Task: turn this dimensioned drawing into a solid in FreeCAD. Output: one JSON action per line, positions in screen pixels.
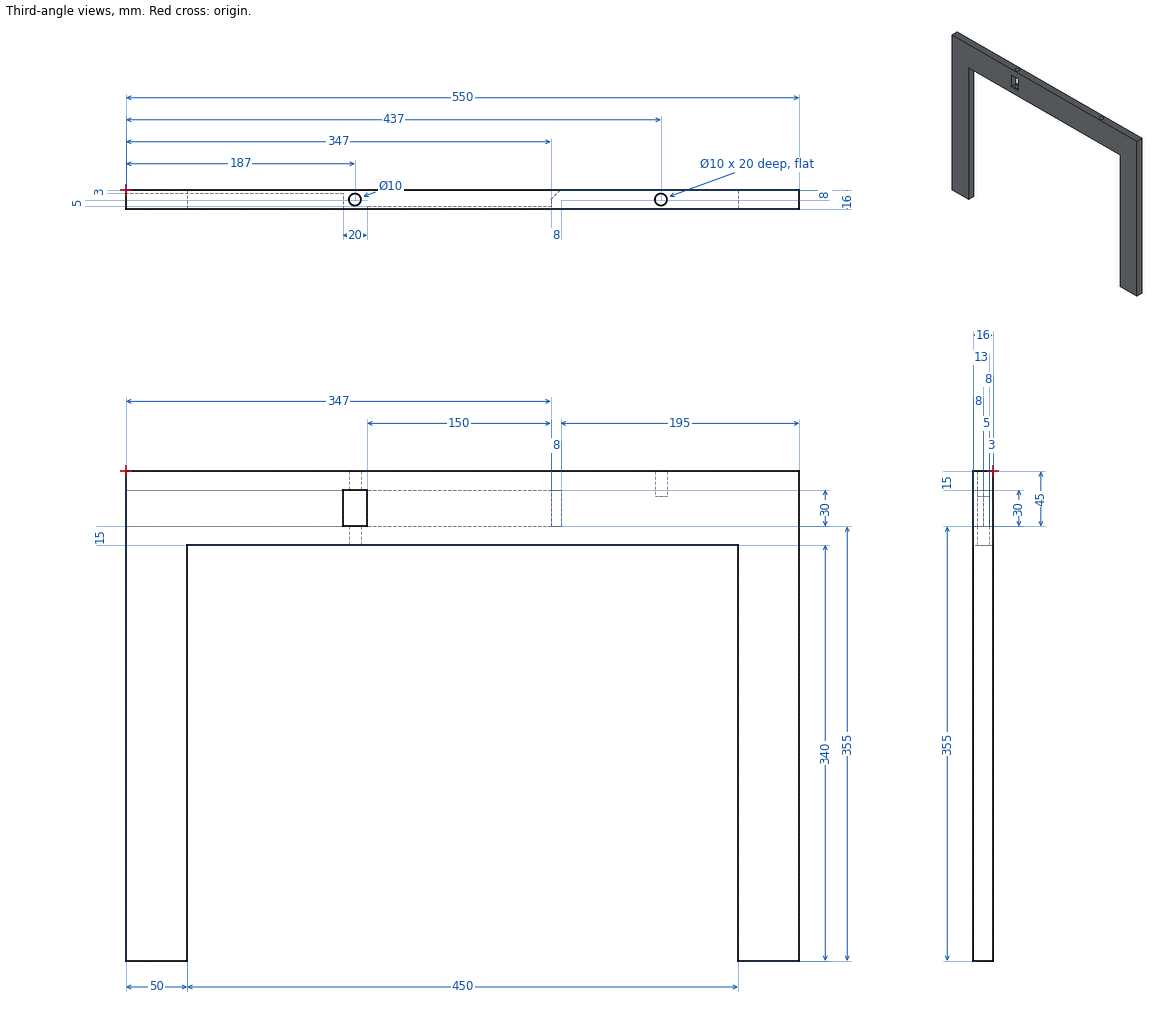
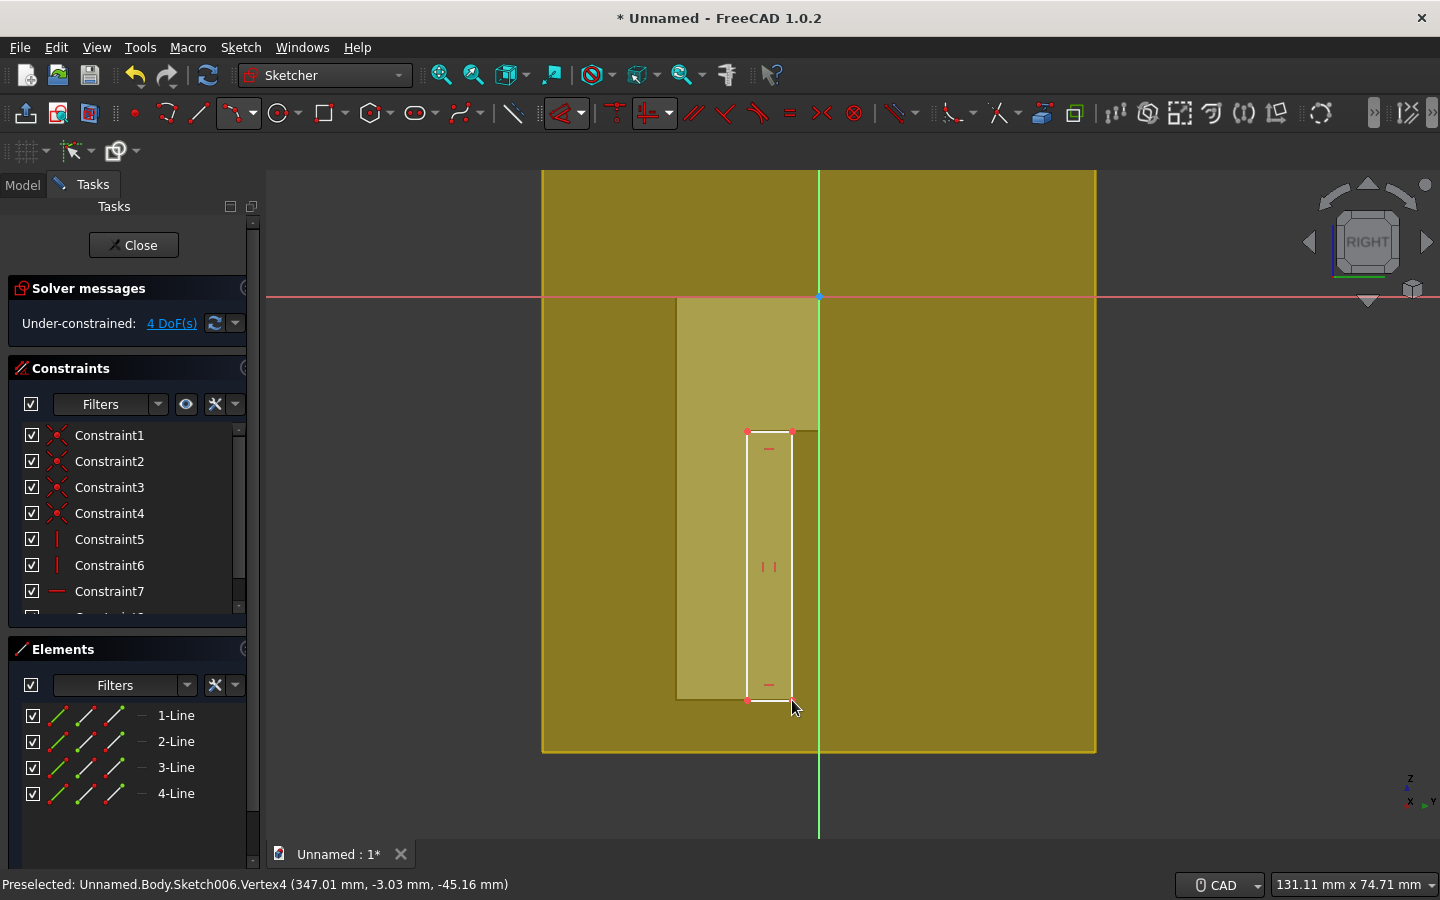
{"action": "left_click", "coordinate": [760, 701]}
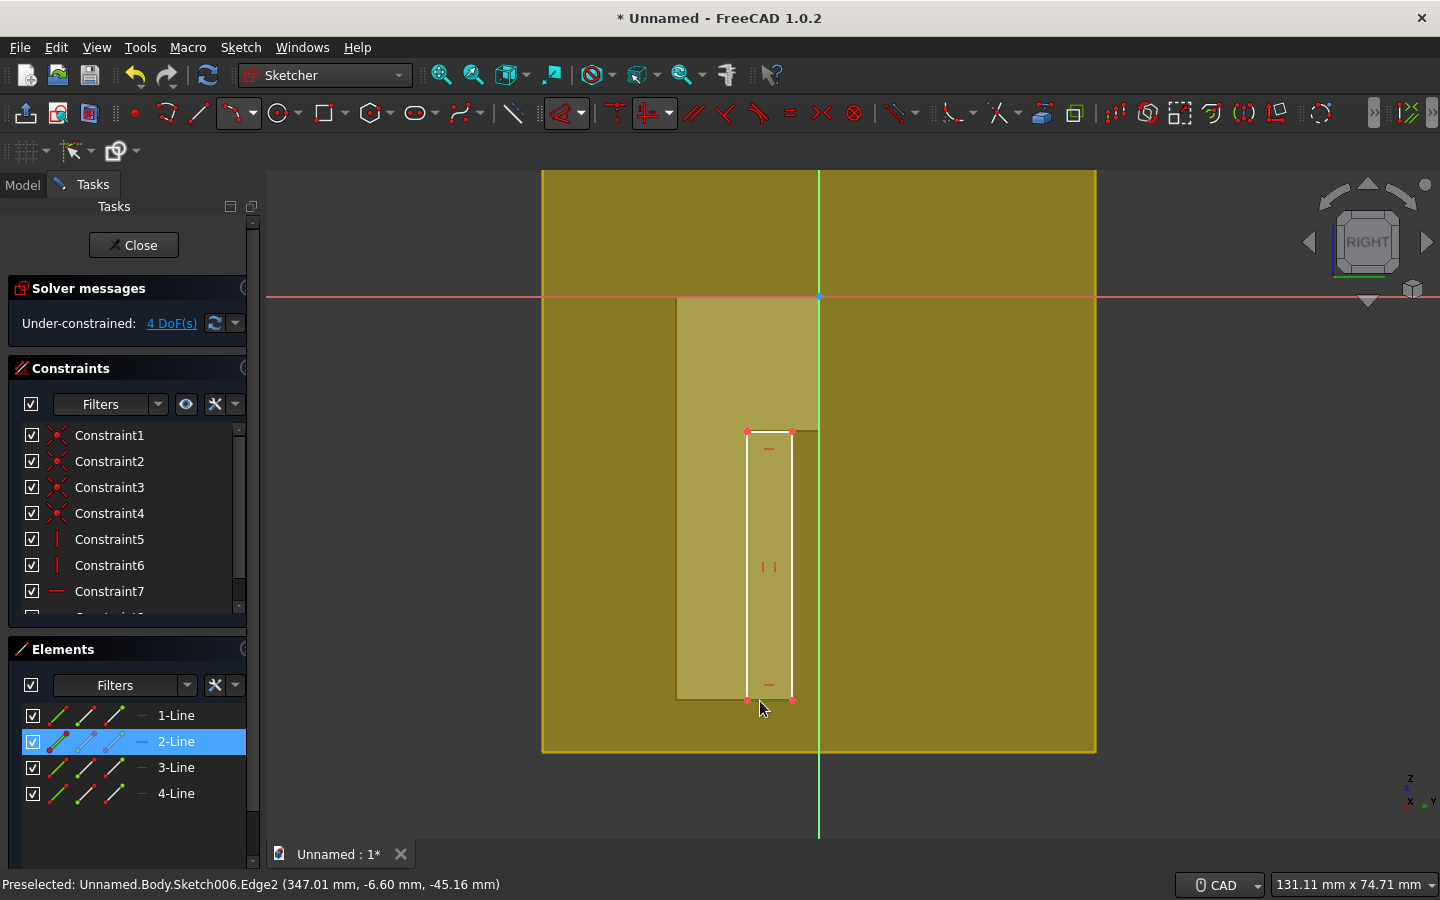
{"action": "key", "text": "l"}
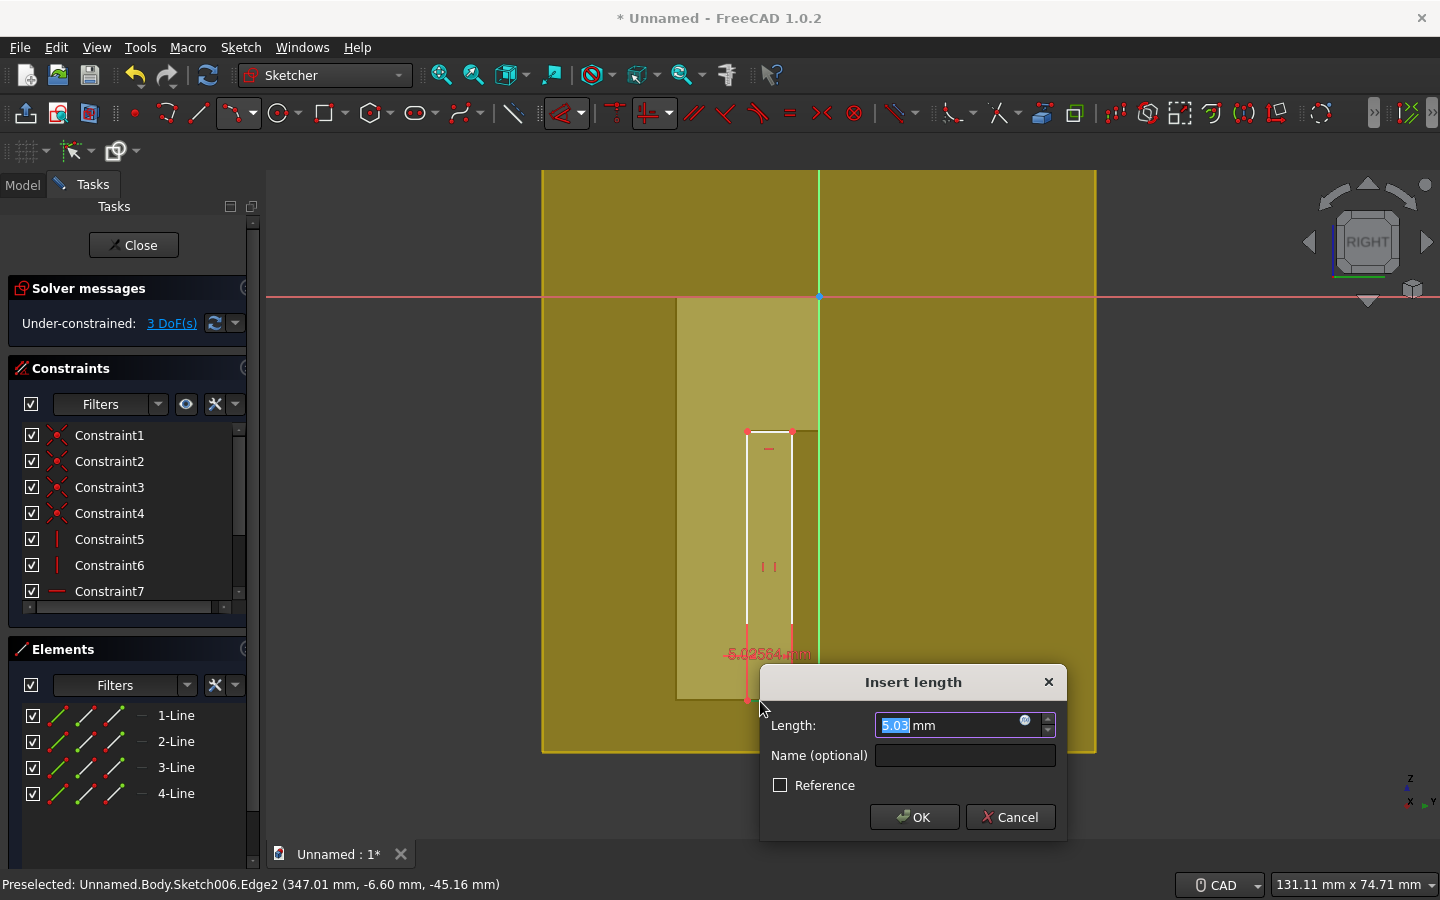
{"action": "type", "text": "5"}
{"action": "key", "text": "Return"}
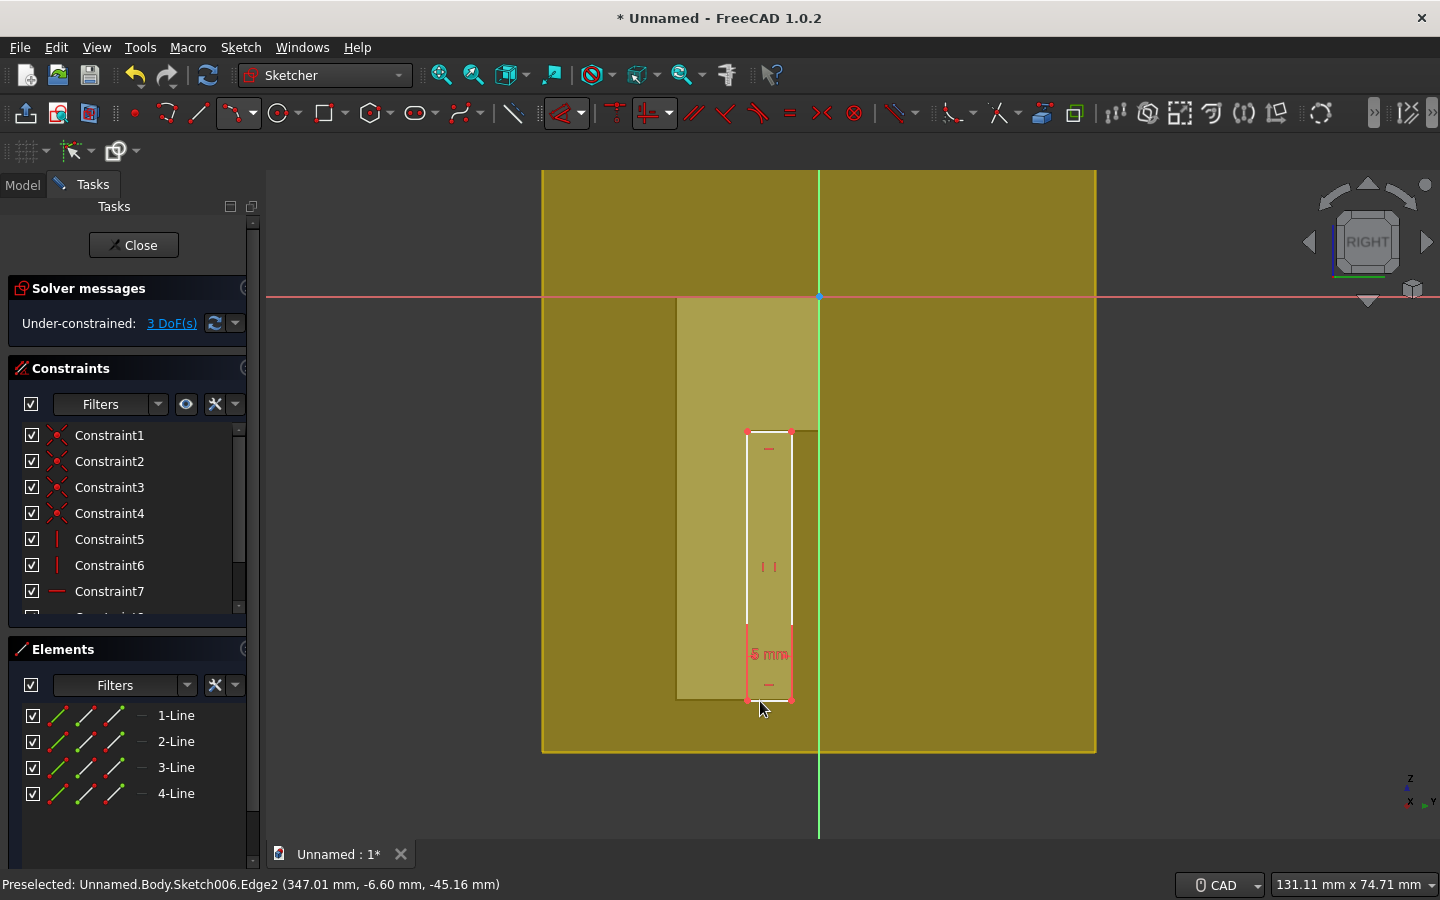
{"action": "left_click", "coordinate": [747, 513]}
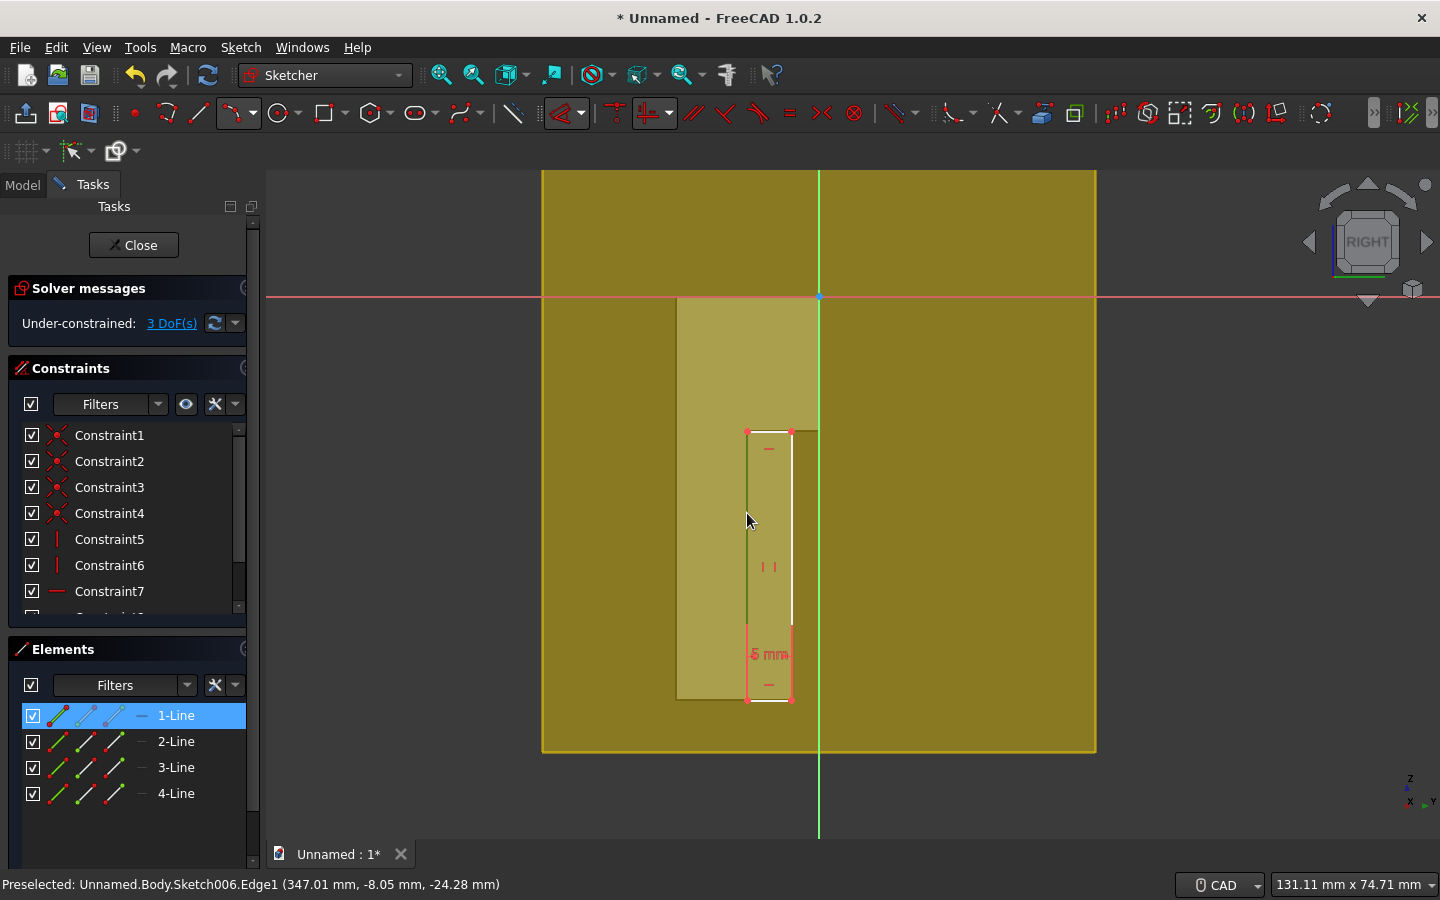
{"action": "left_click", "coordinate": [584, 114]}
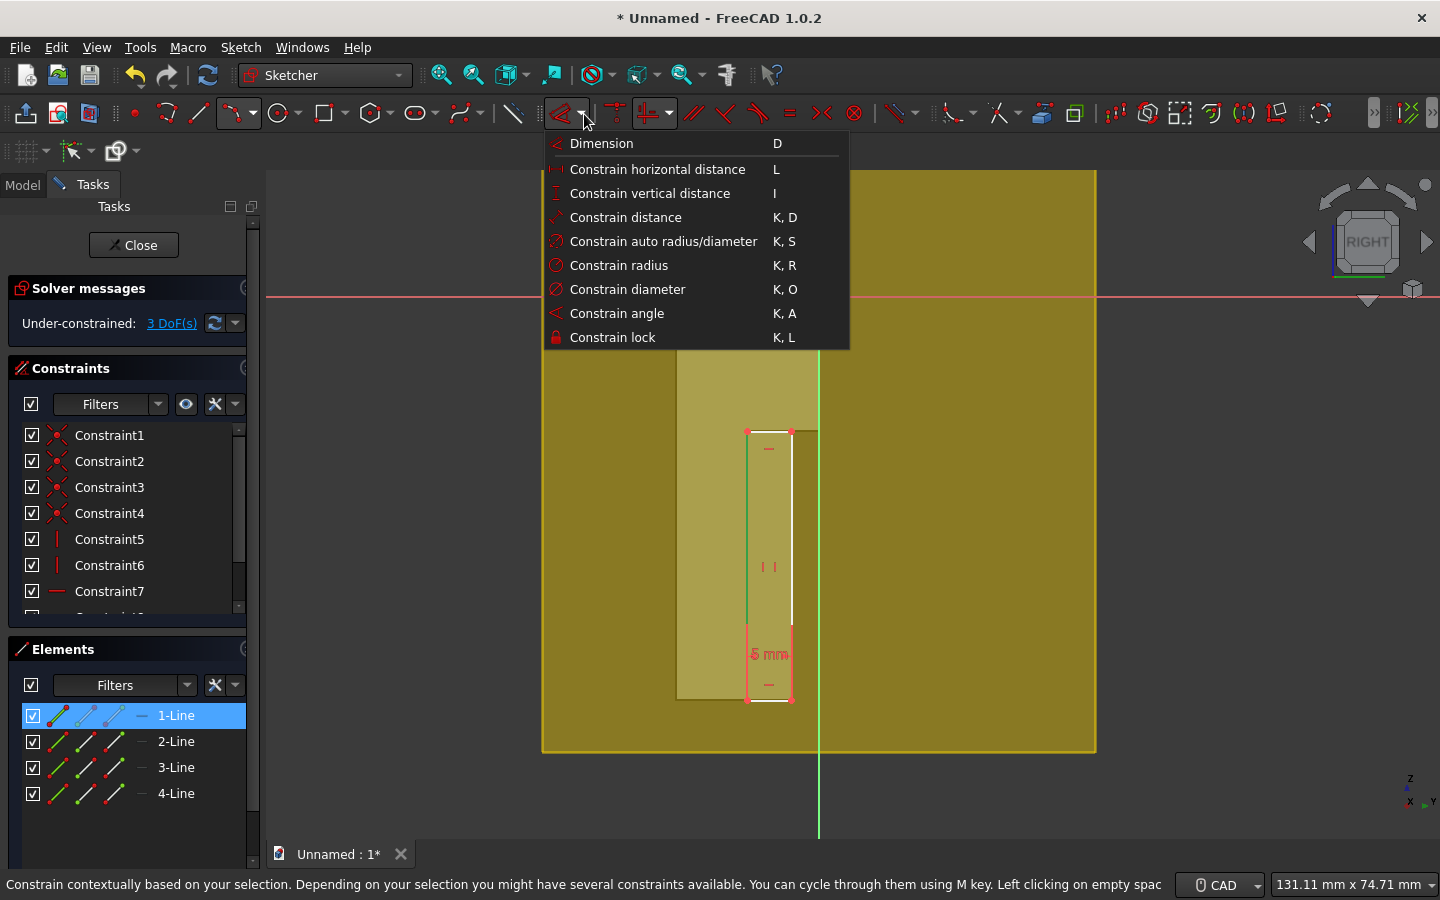
{"action": "left_click", "coordinate": [697, 193]}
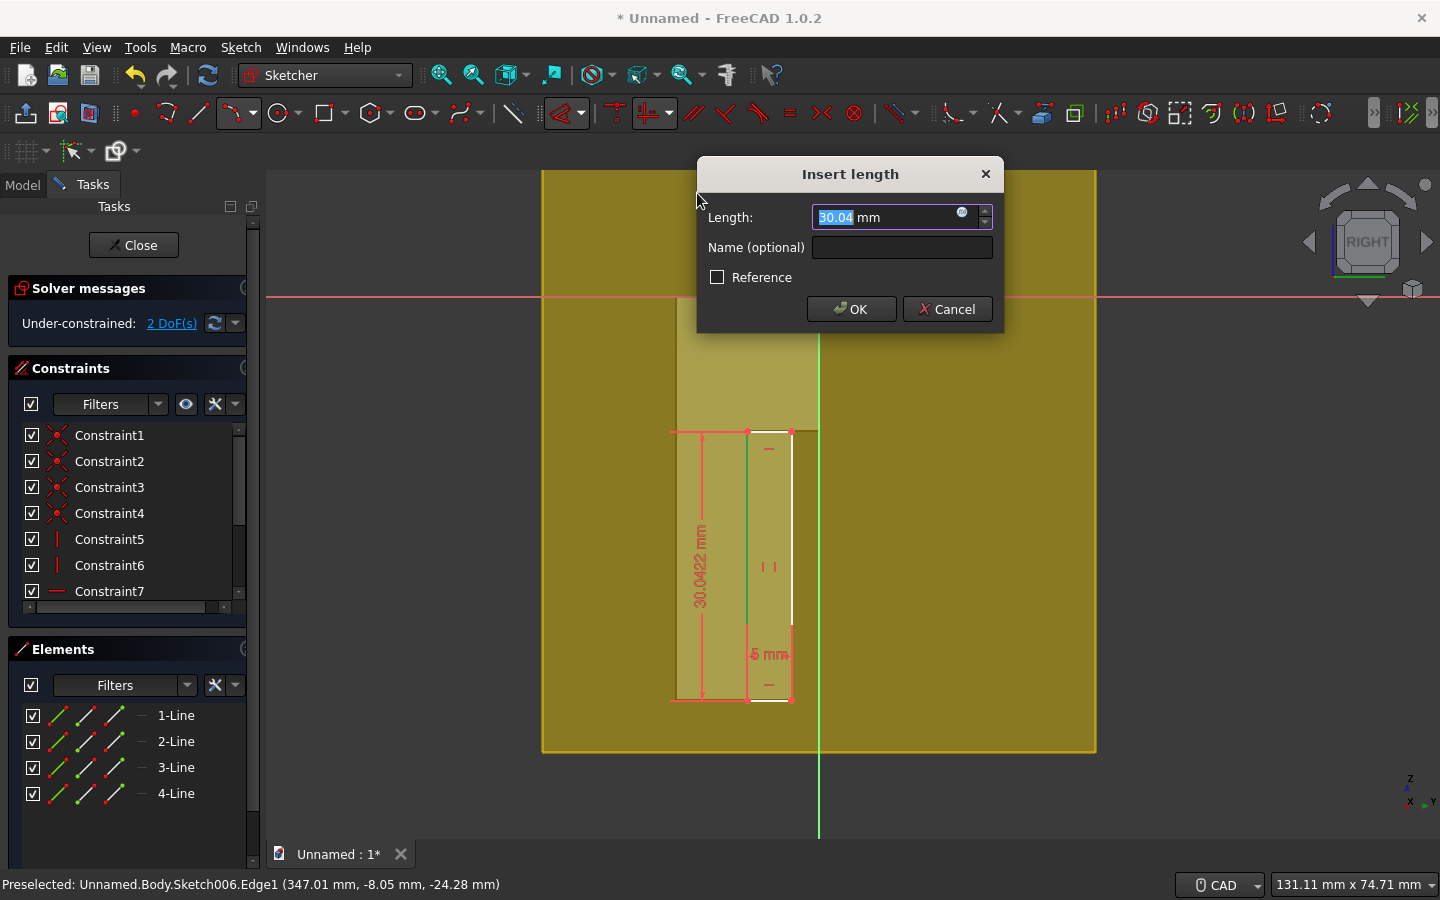
{"action": "type", "text": "30"}
{"action": "key", "text": "Return"}